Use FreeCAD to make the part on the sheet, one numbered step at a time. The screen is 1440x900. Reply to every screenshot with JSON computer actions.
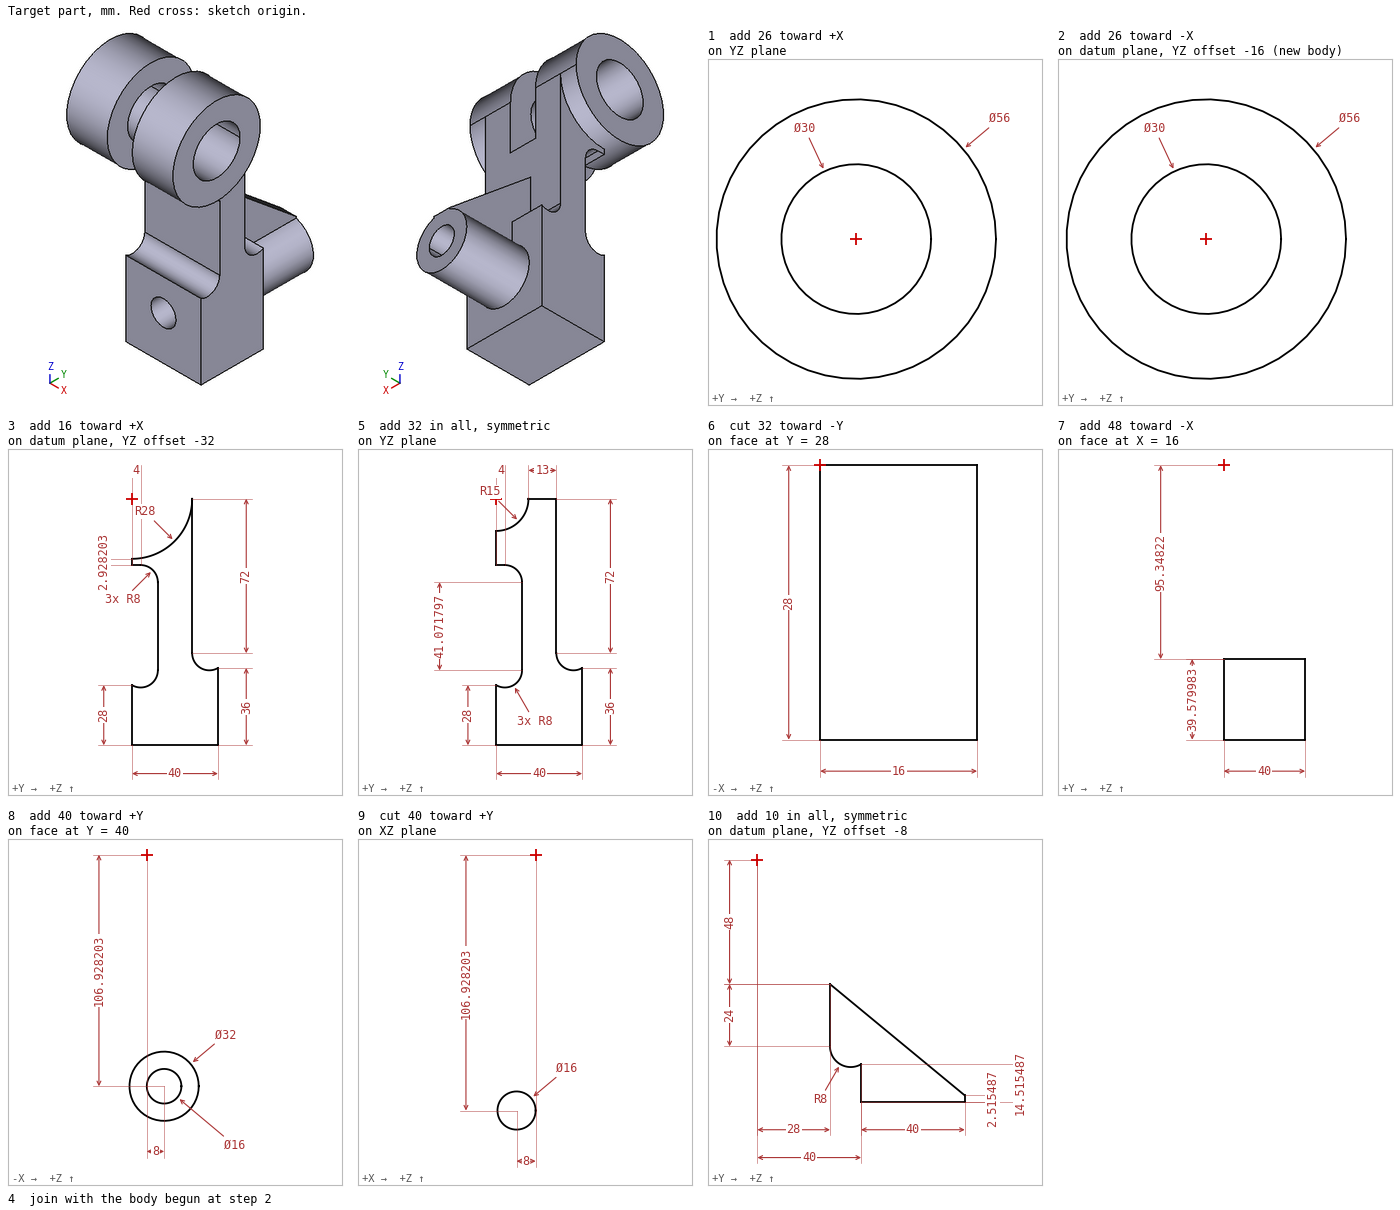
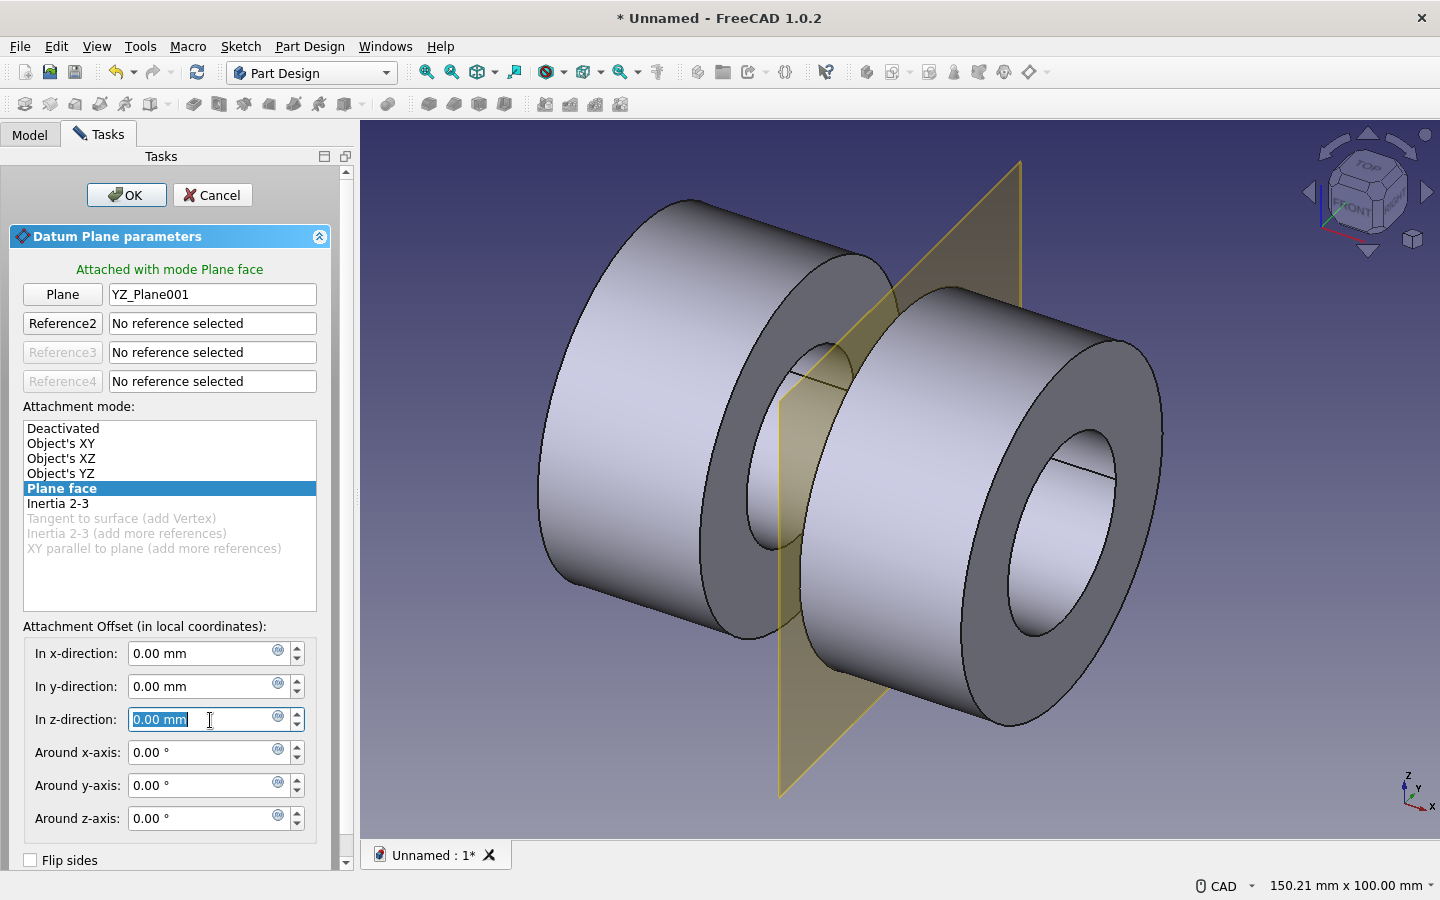
{"action": "type", "text": "-32"}
{"action": "key", "text": "Tab"}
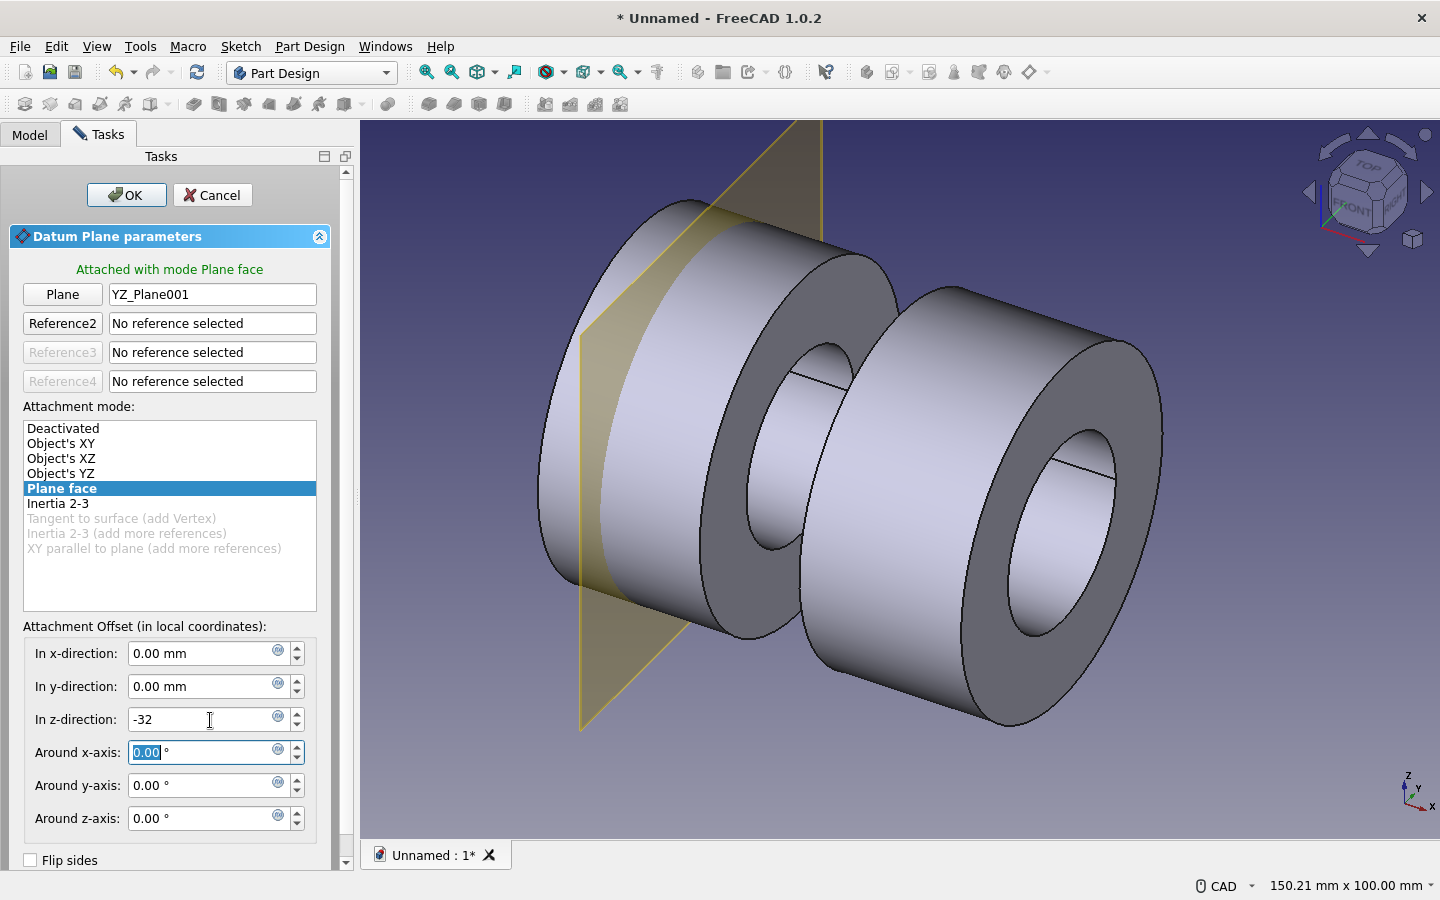
{"action": "left_click", "coordinate": [127, 195]}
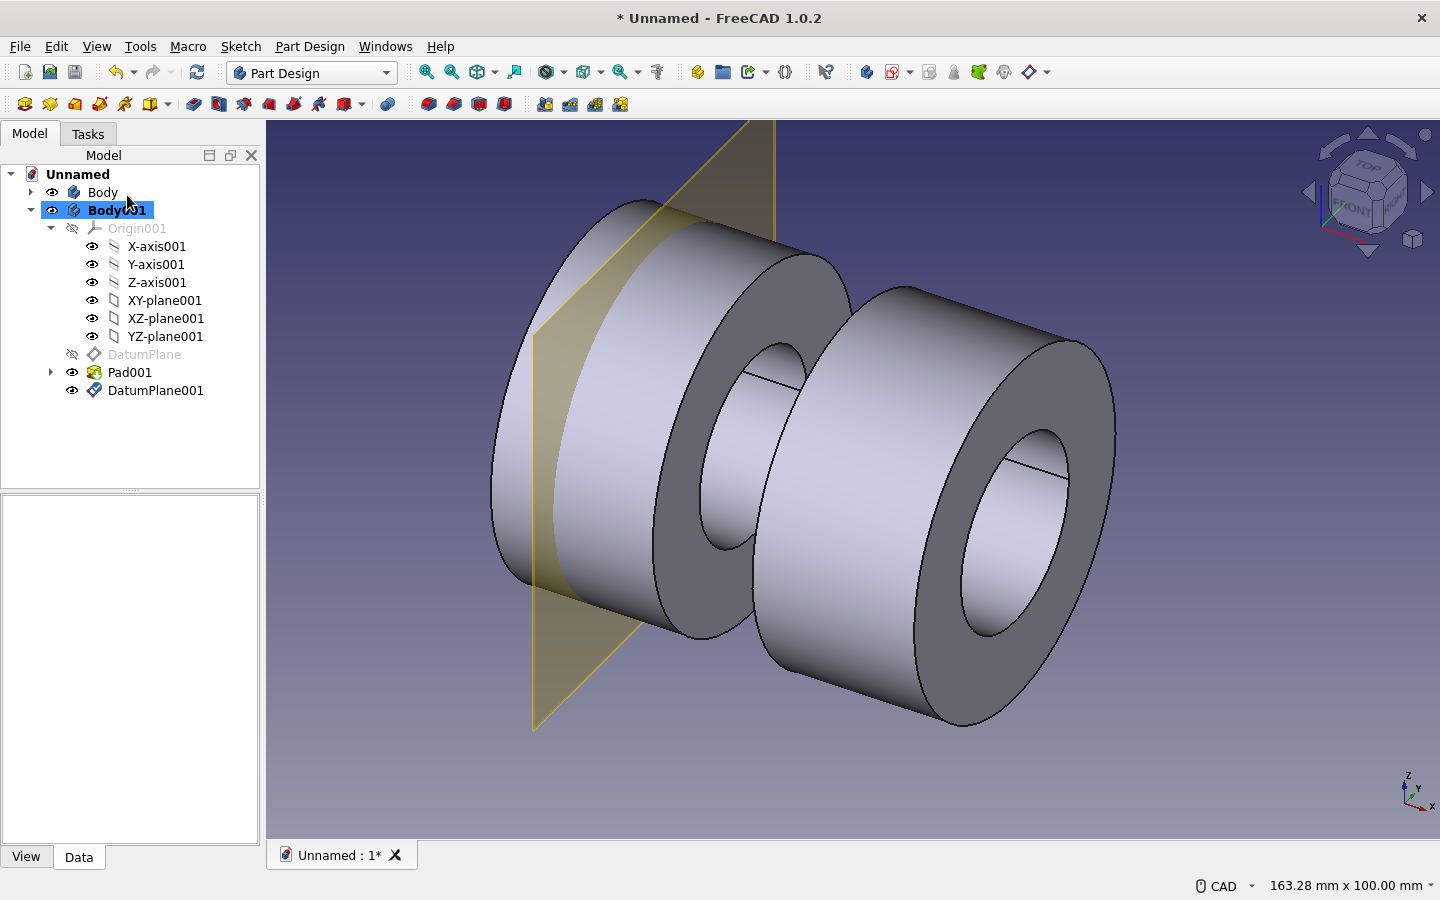
{"action": "left_click", "coordinate": [117, 390]}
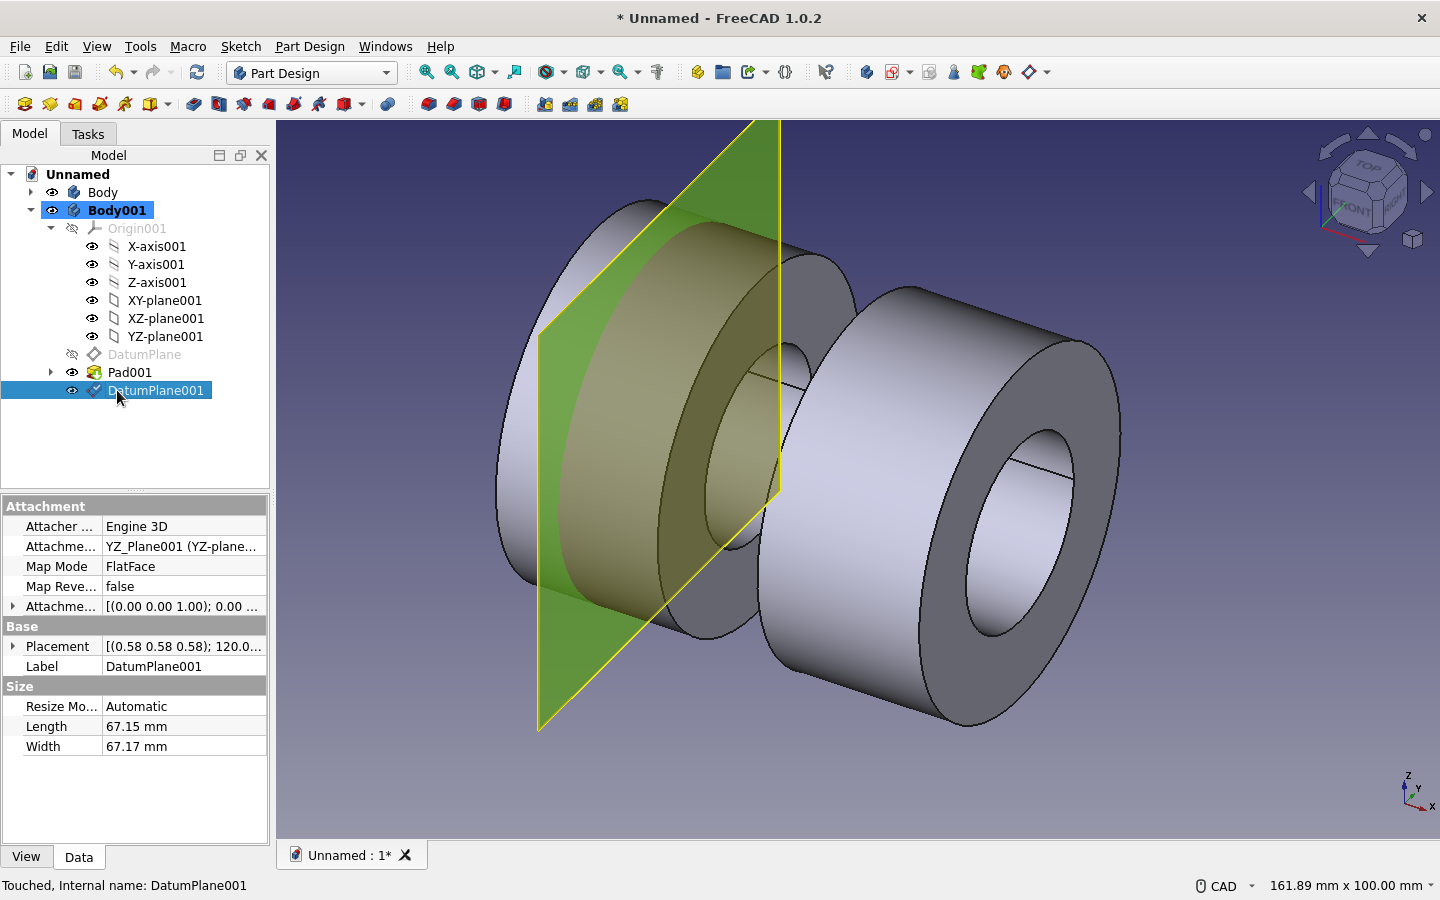
{"action": "left_click", "coordinate": [892, 72]}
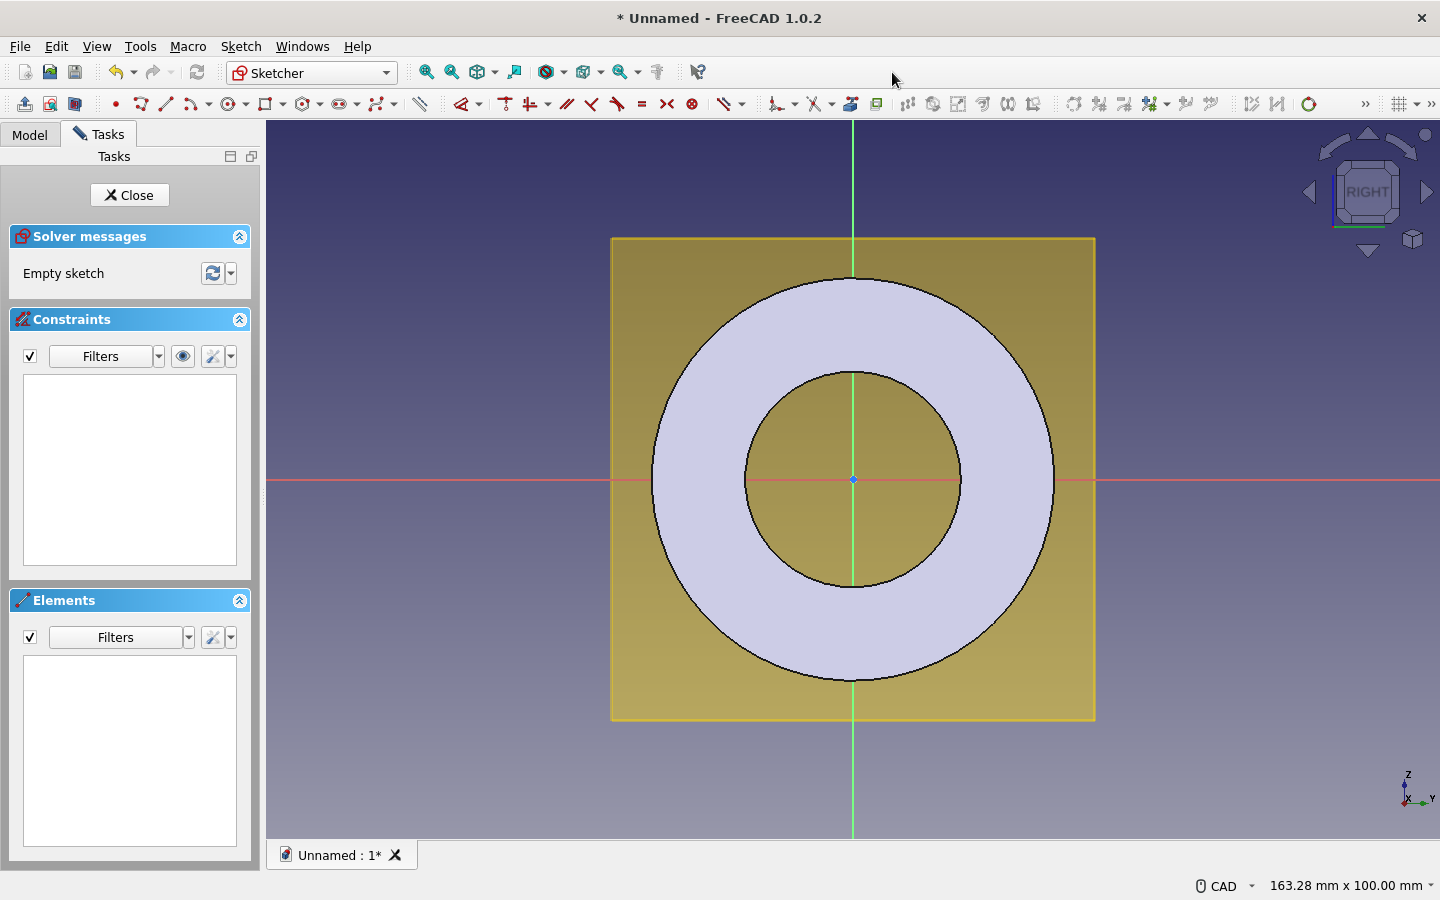
{"action": "key", "text": "q s"}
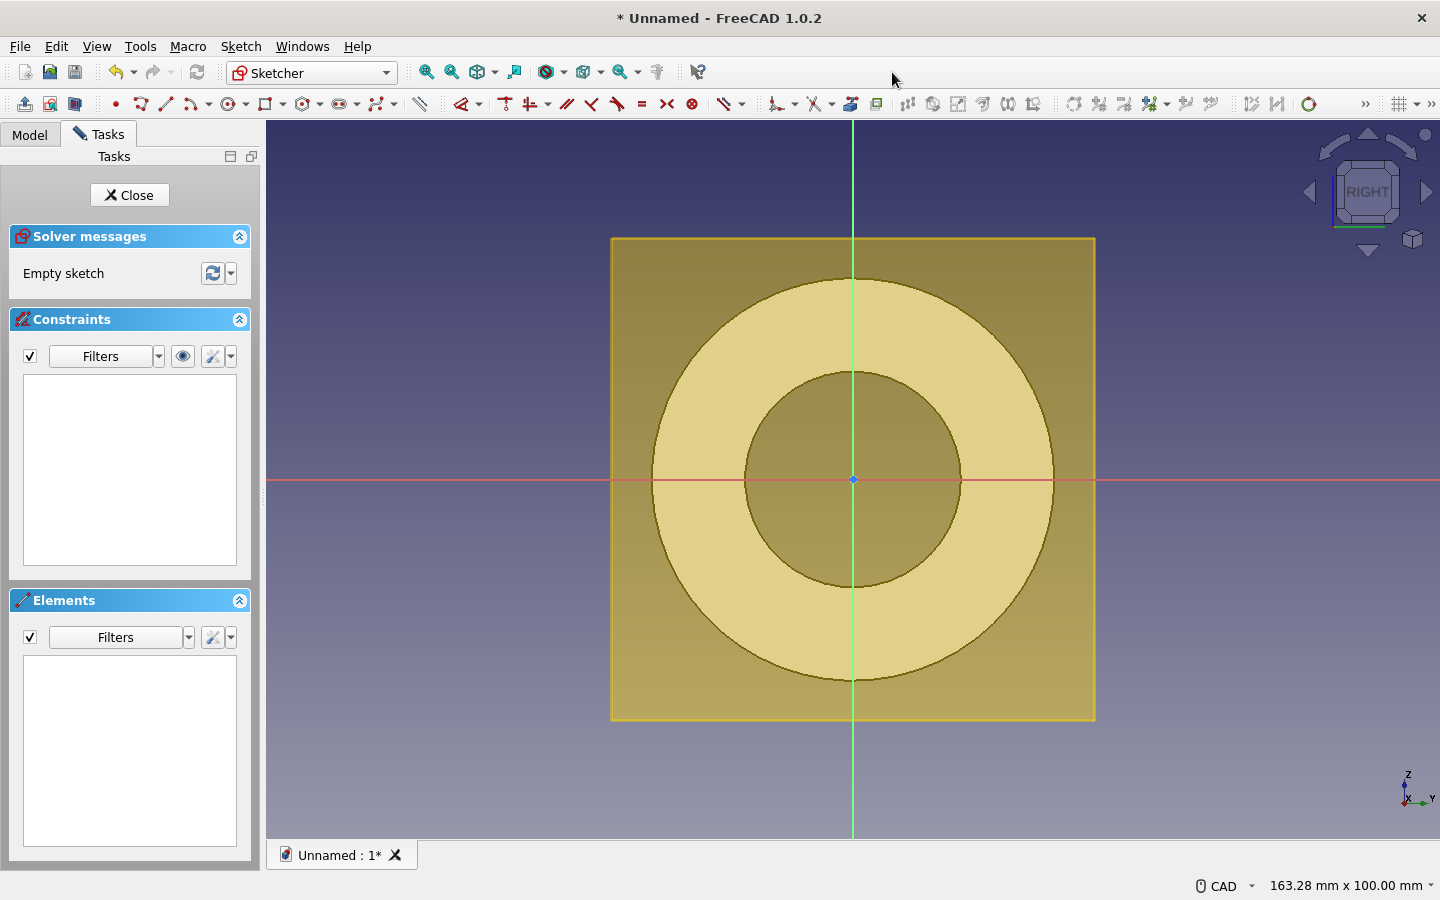
{"action": "scroll", "coordinate": [526, 148], "scroll_direction": "down", "scroll_amount": 3}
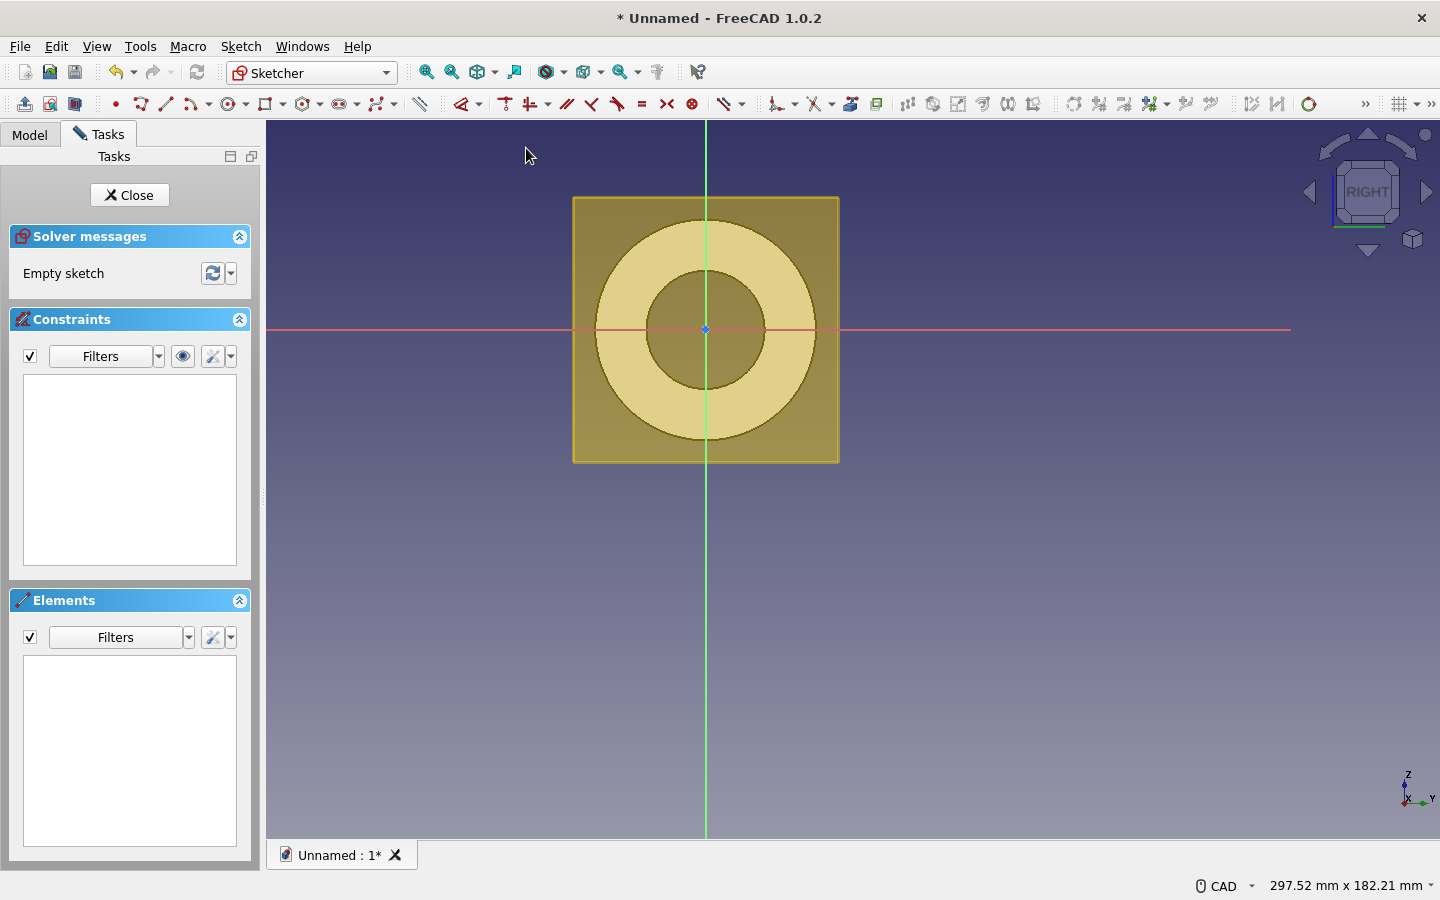
{"action": "key", "text": "g l"}